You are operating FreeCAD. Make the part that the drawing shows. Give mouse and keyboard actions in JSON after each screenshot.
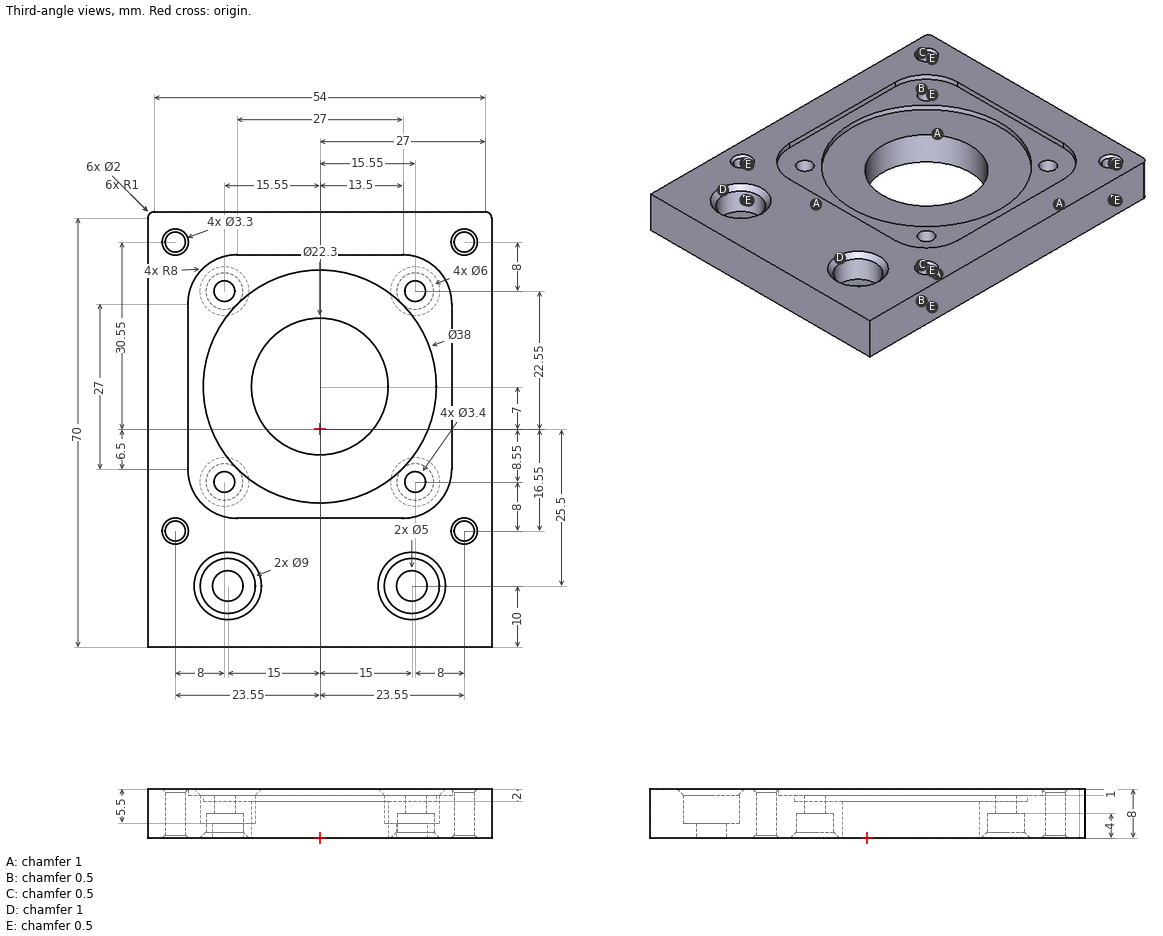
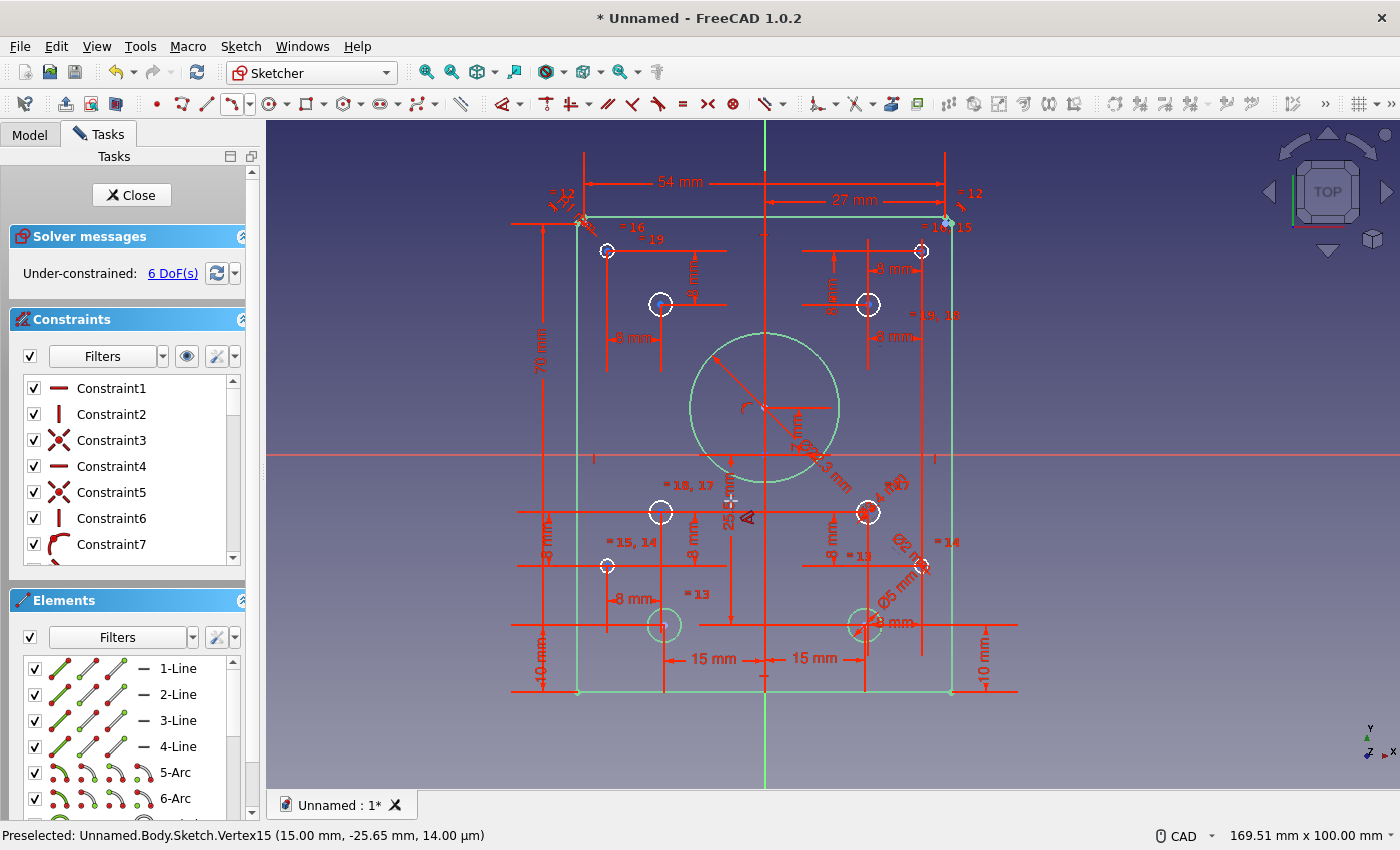
{"action": "left_click", "coordinate": [868, 512]}
{"action": "left_click", "coordinate": [902, 470]}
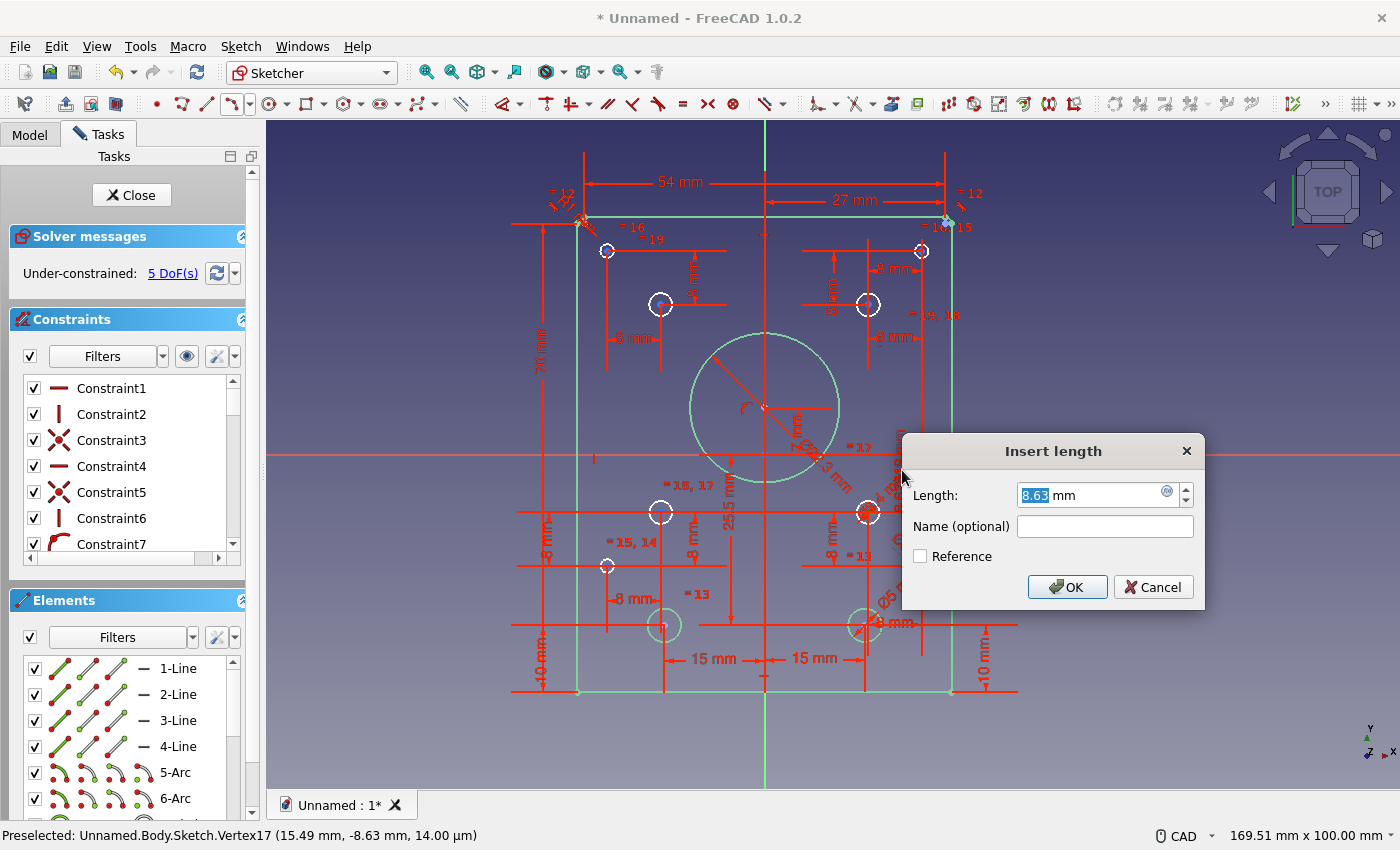
{"action": "type", "text": "8.55"}
{"action": "key", "text": "Return"}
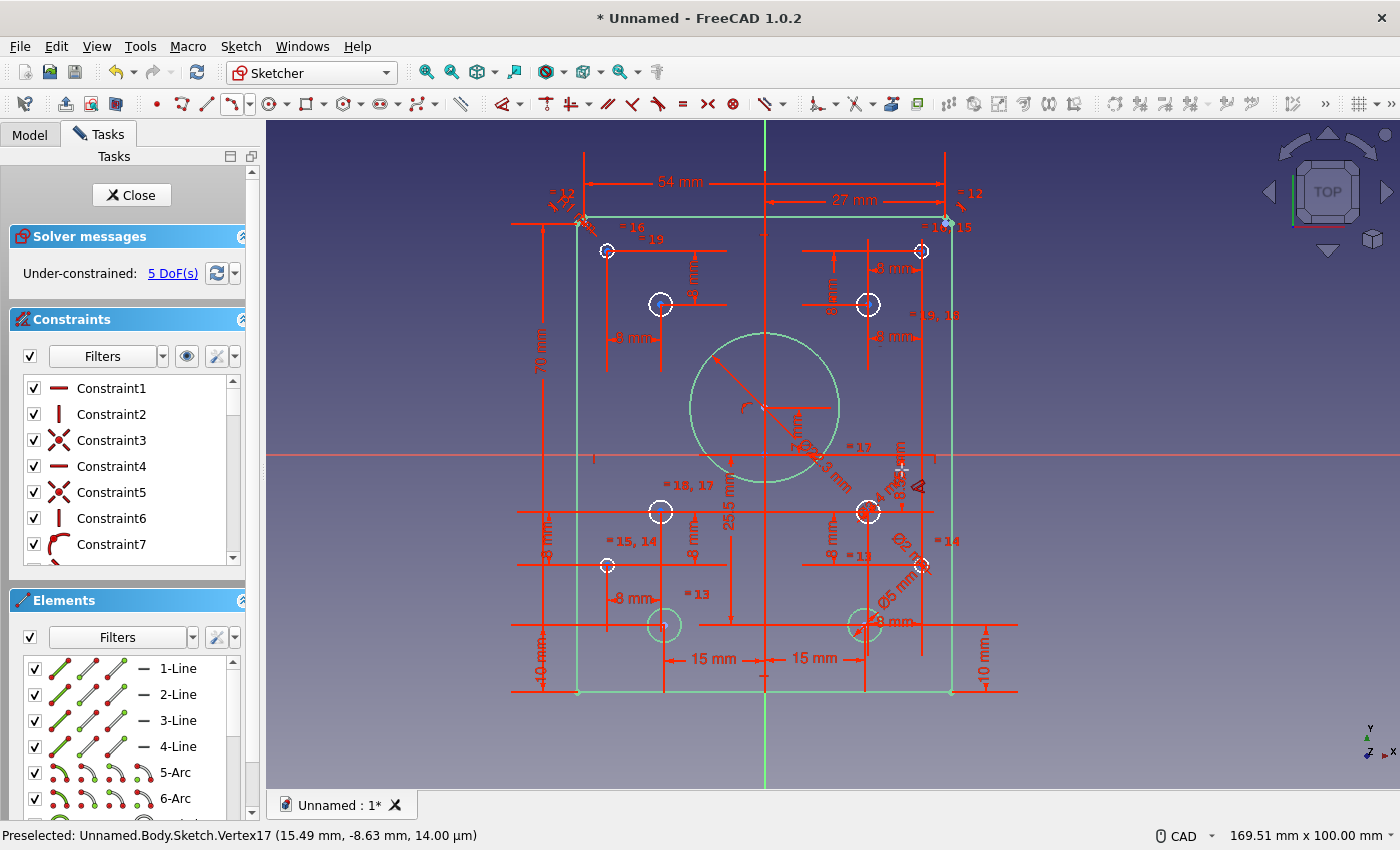
{"action": "left_click", "coordinate": [922, 565]}
{"action": "left_click", "coordinate": [807, 599]}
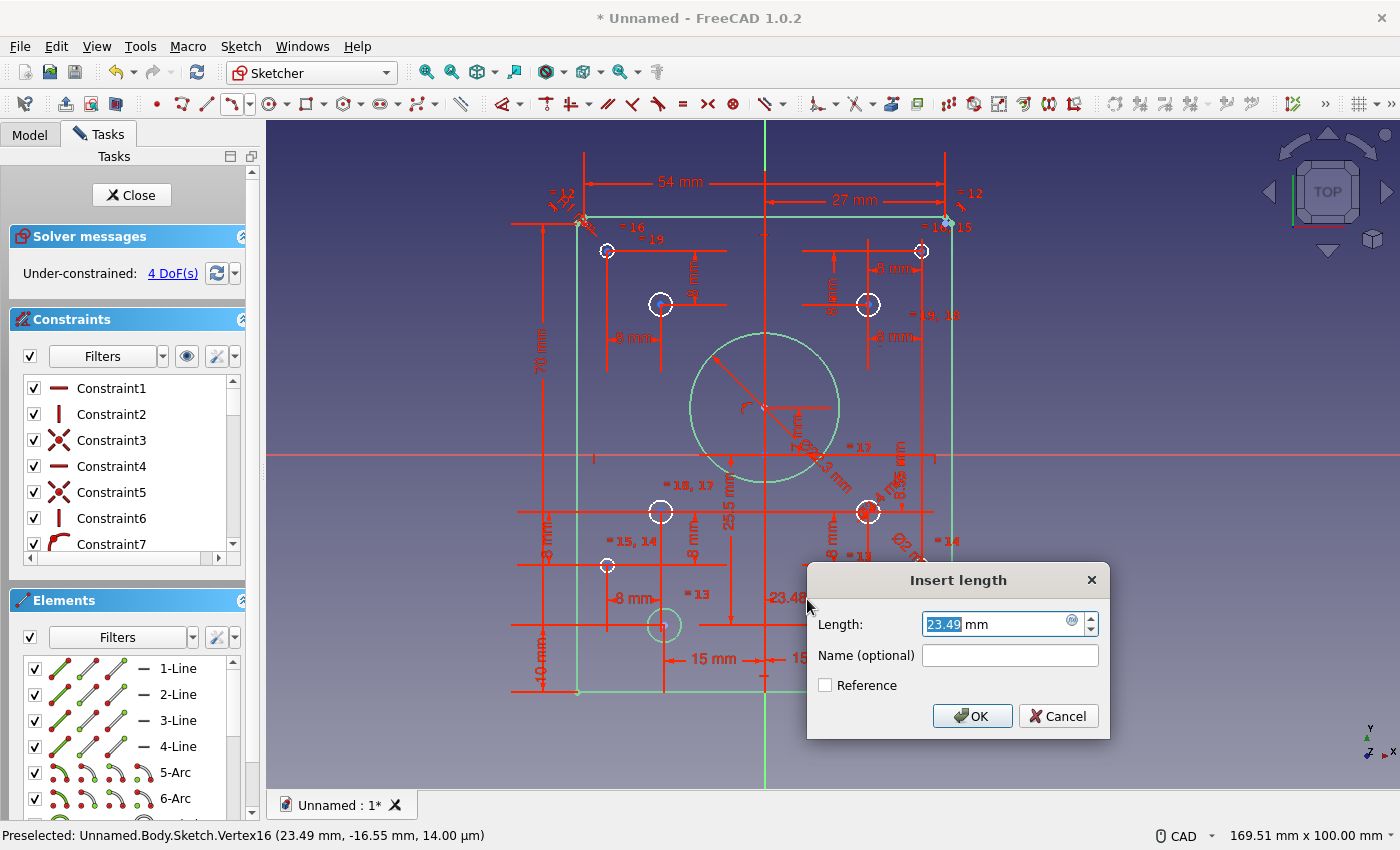
{"action": "type", "text": "23.55"}
{"action": "key", "text": "Return"}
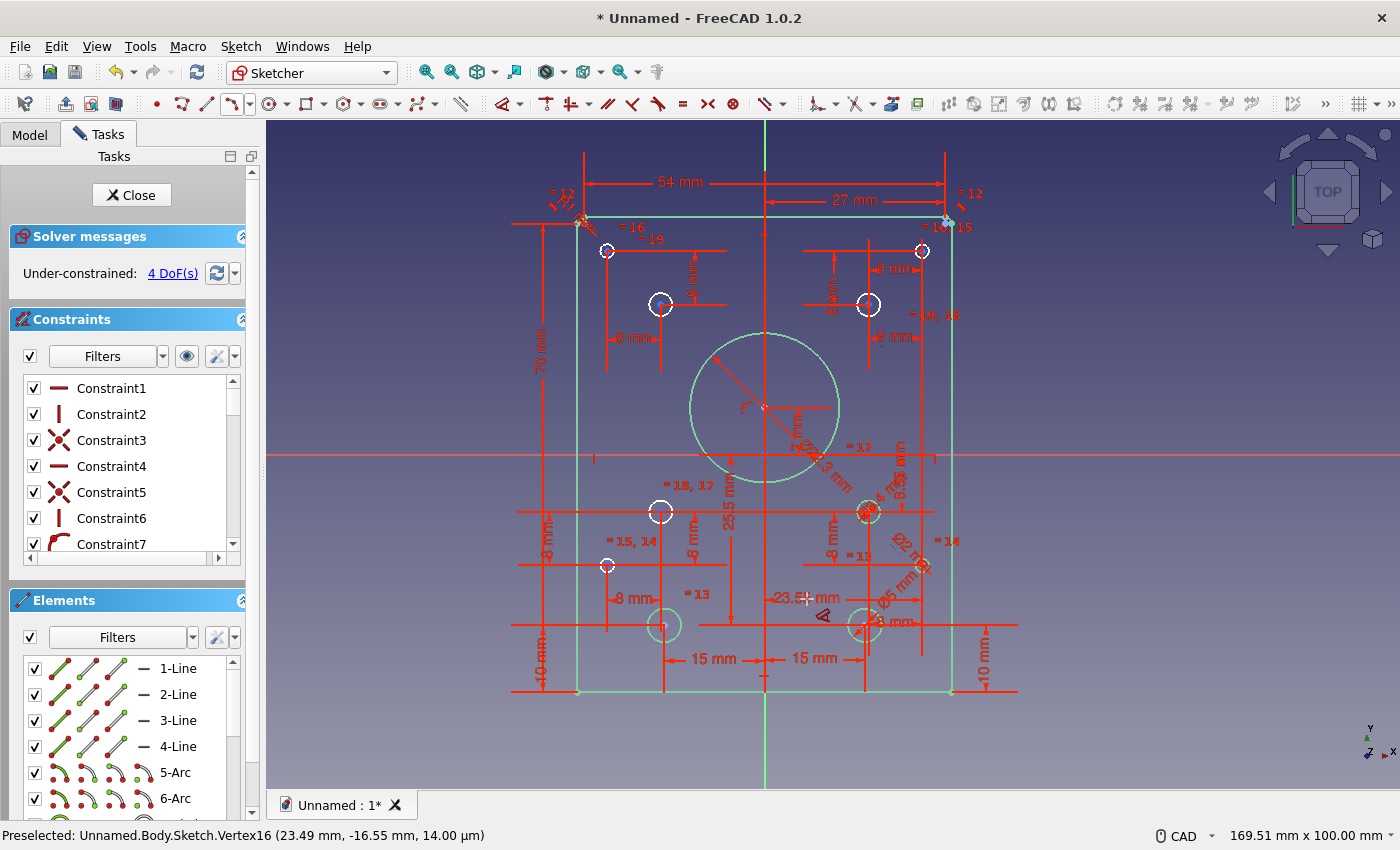
{"action": "left_click", "coordinate": [607, 565]}
{"action": "left_click", "coordinate": [722, 599]}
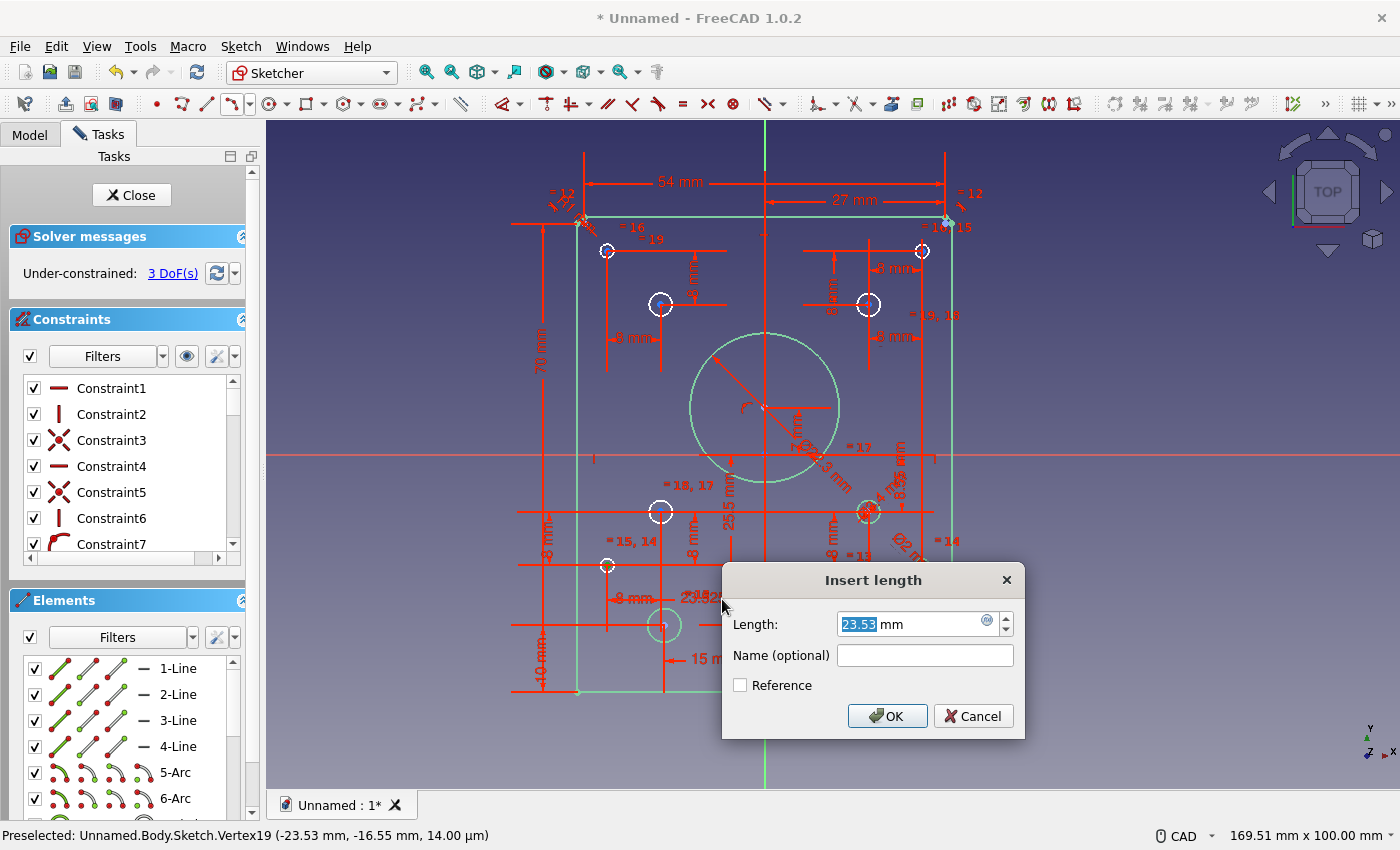
{"action": "type", "text": "23.55"}
{"action": "key", "text": "Return"}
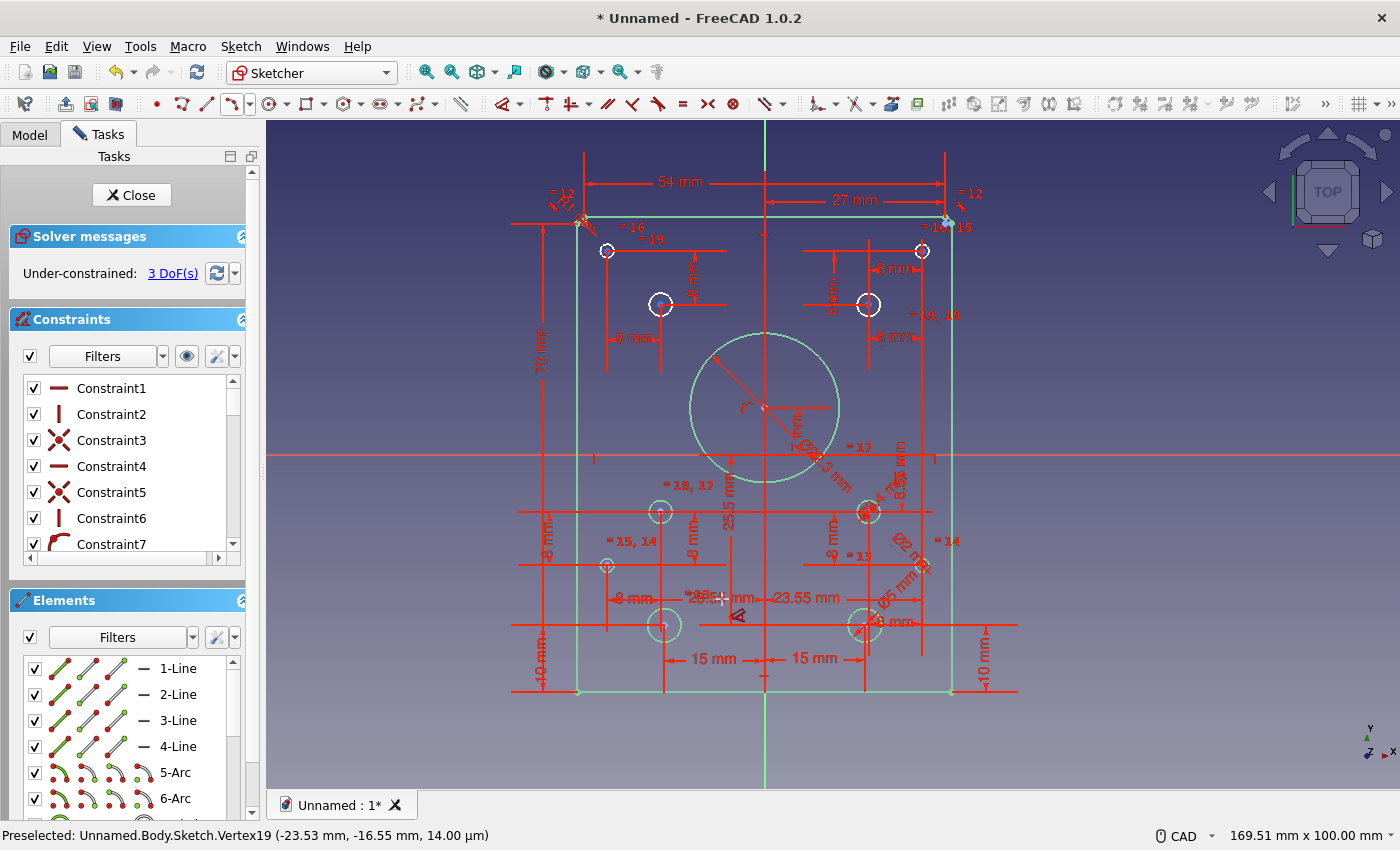
{"action": "left_click", "coordinate": [869, 305]}
{"action": "left_click", "coordinate": [903, 380]}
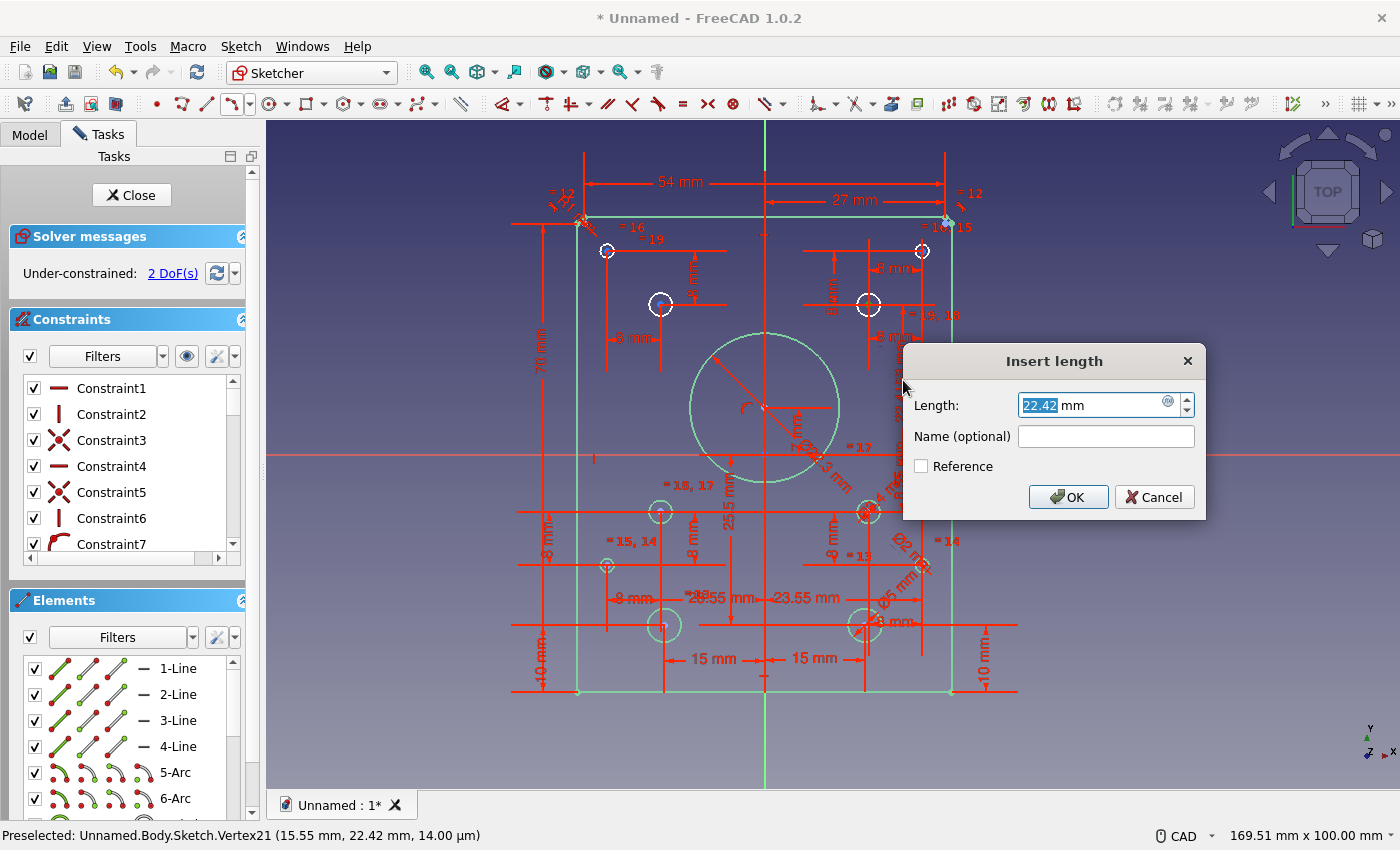
{"action": "type", "text": "22.55"}
{"action": "key", "text": "Return"}